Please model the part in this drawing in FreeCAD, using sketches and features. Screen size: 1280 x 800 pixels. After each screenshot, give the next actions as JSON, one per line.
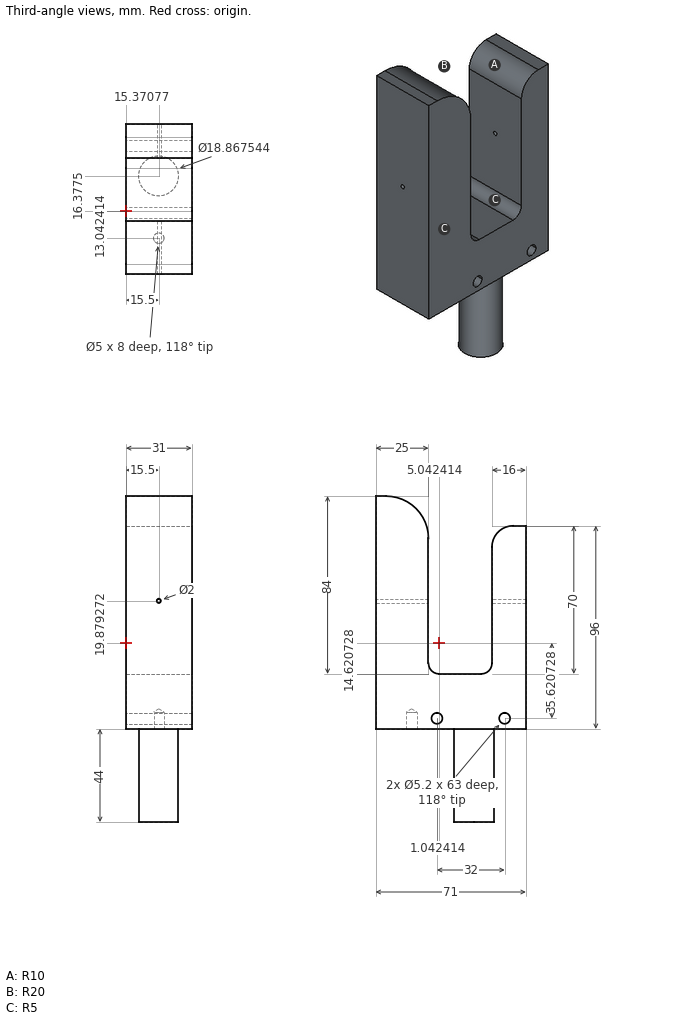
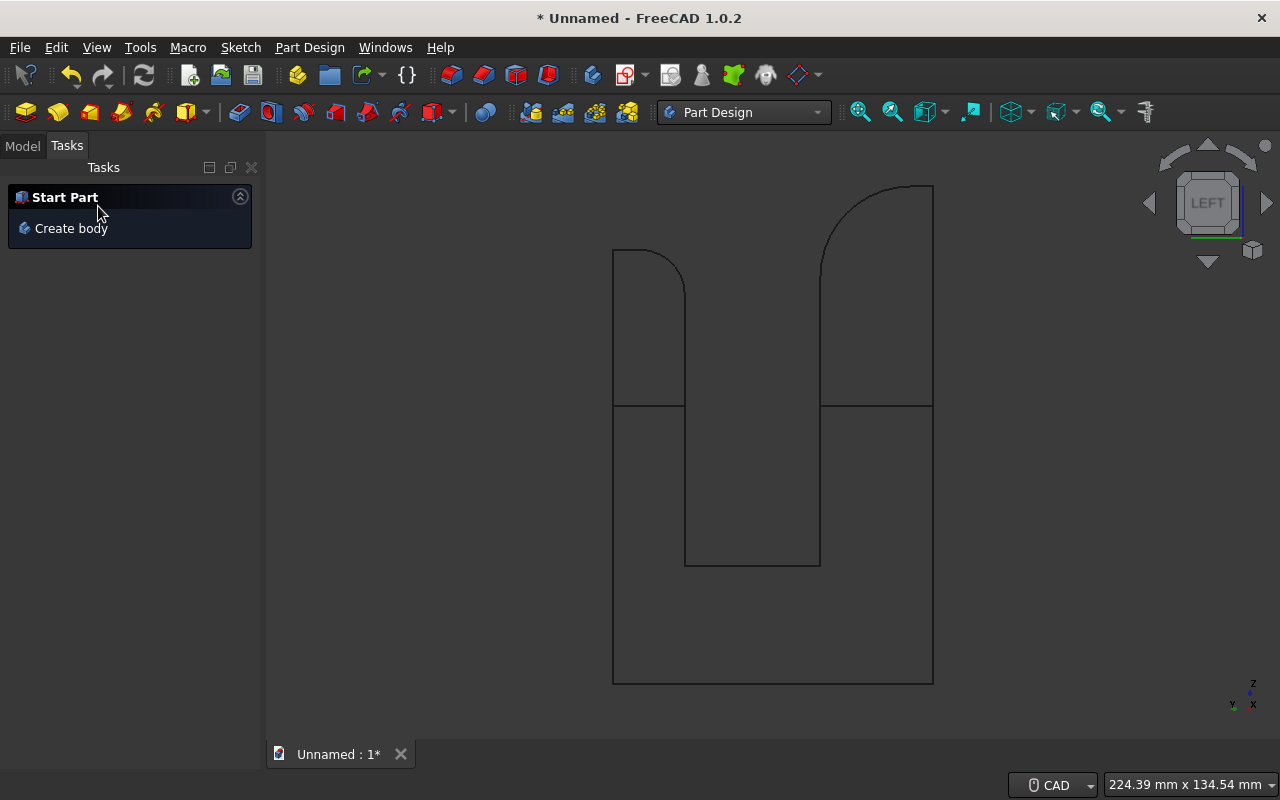
{"action": "key", "text": "0"}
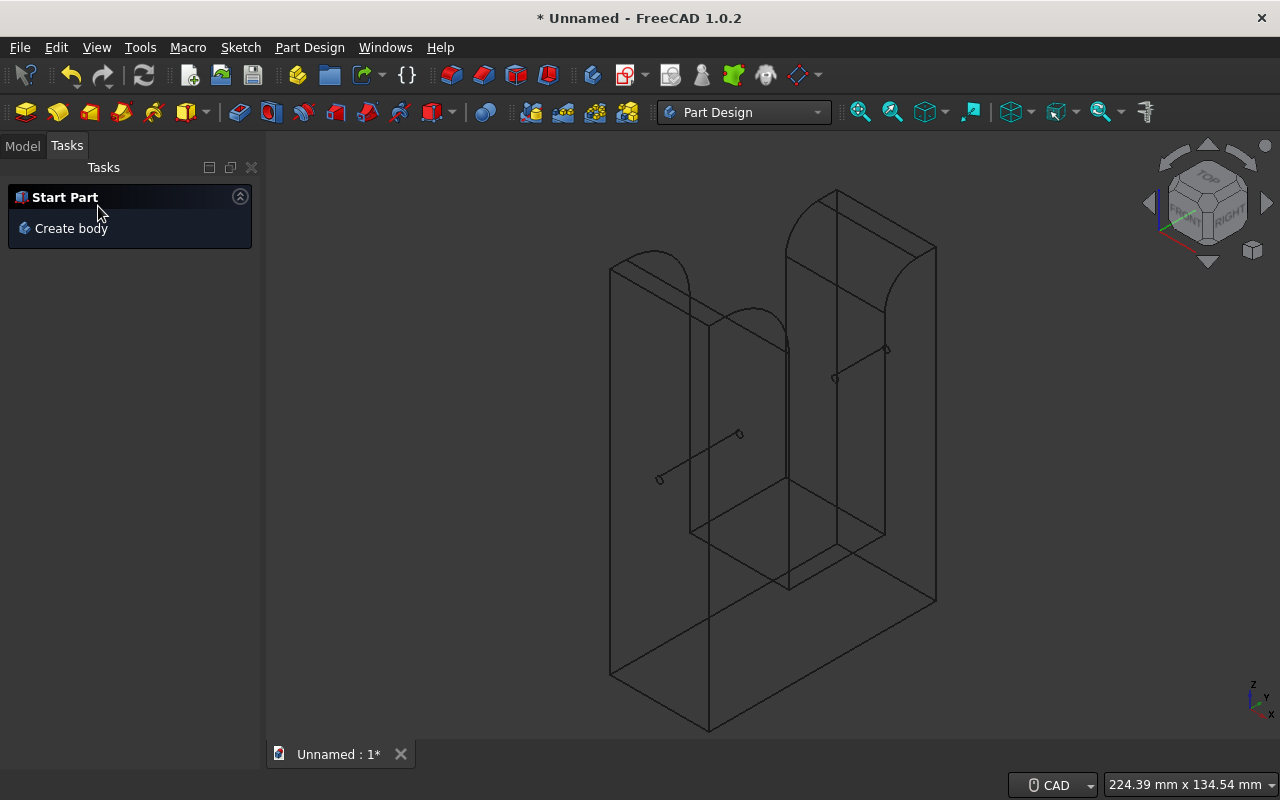
{"action": "left_click", "coordinate": [739, 560]}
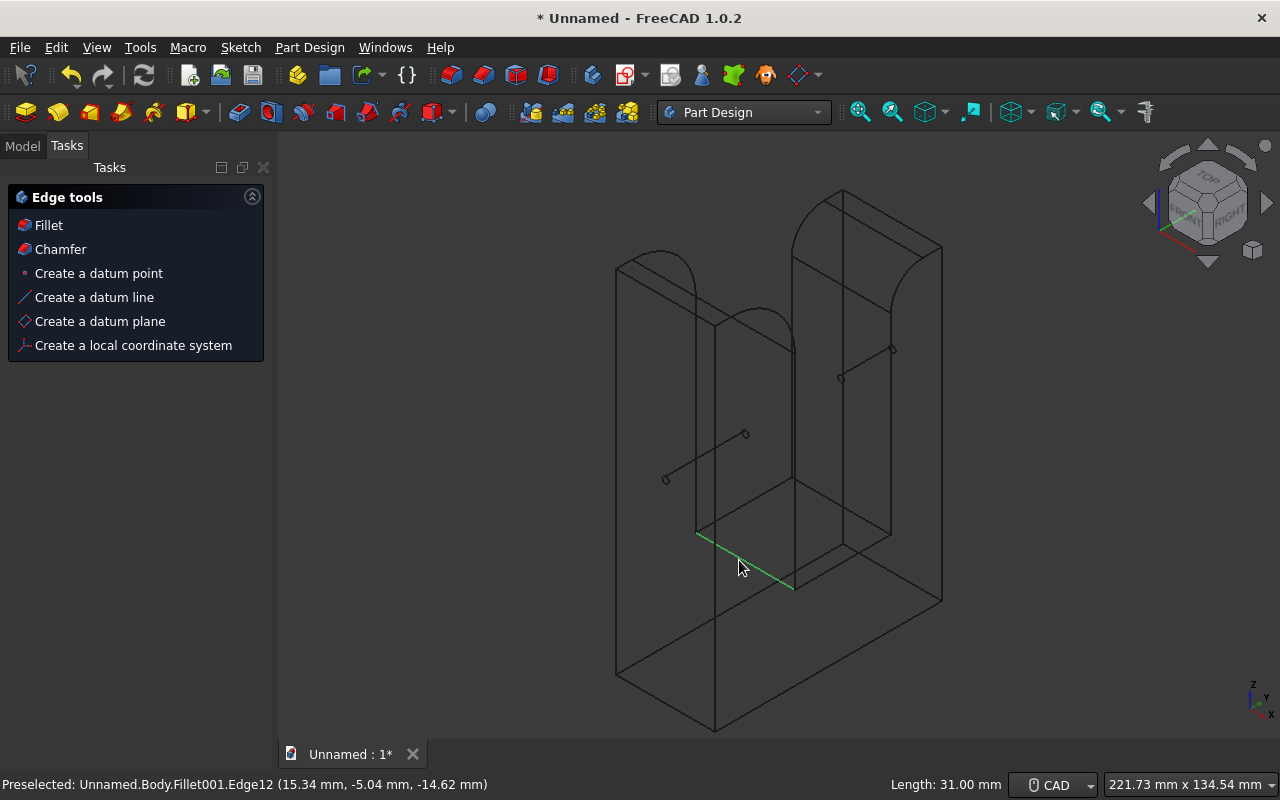
{"action": "left_click", "coordinate": [841, 505], "text": "ctrl"}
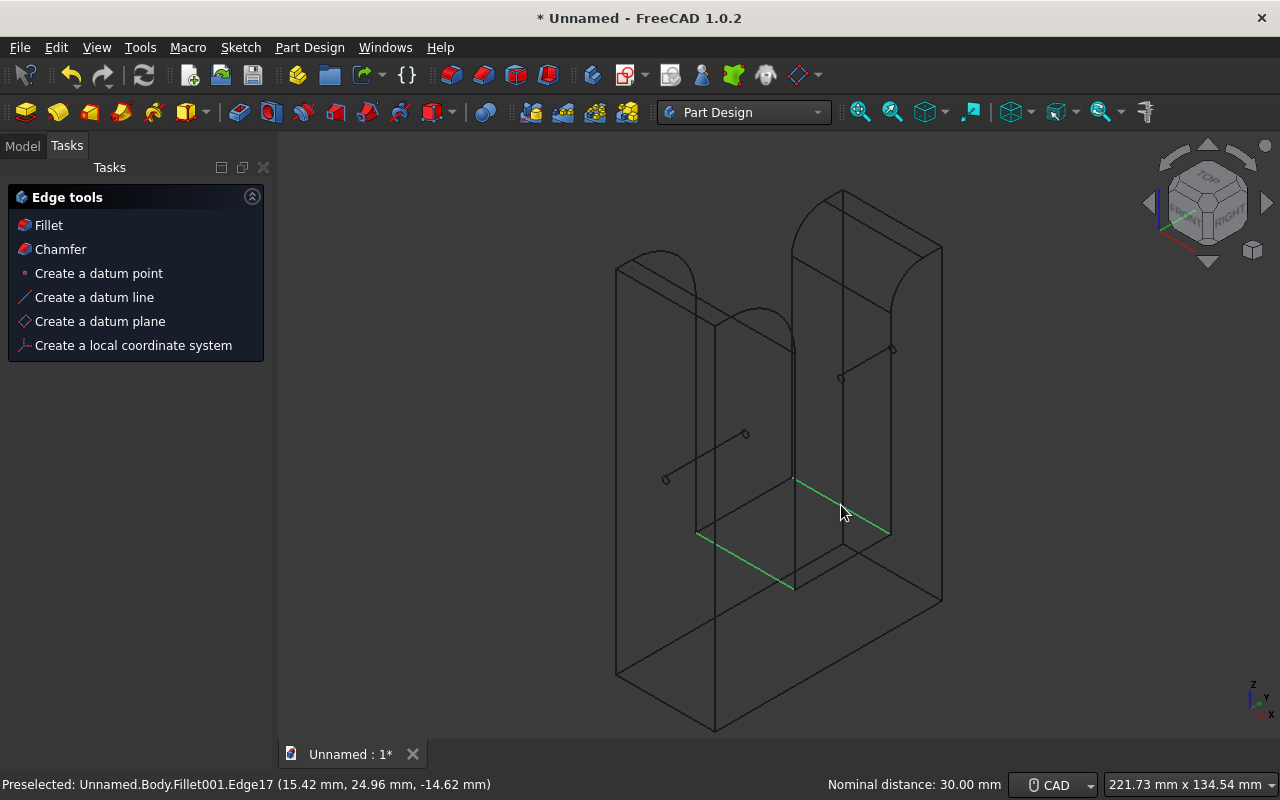
{"action": "key", "text": "v 1"}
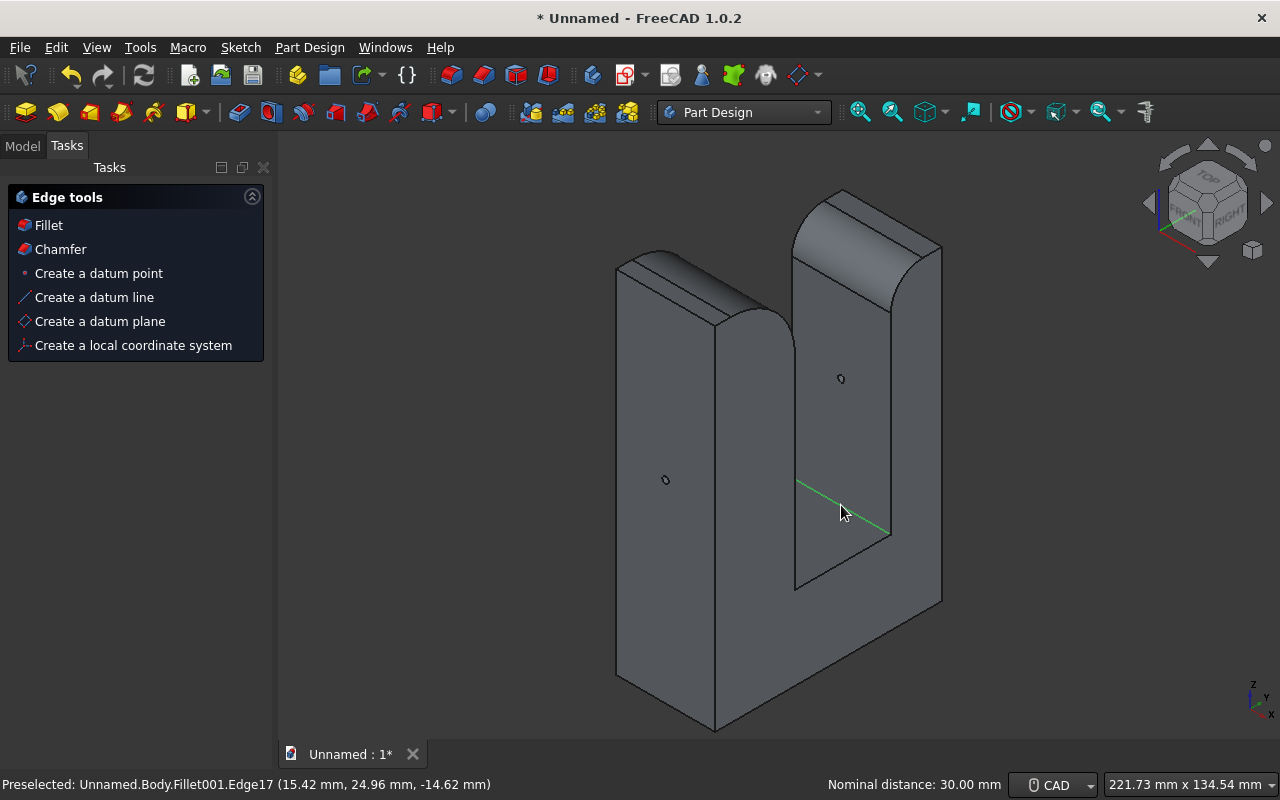
{"action": "left_click", "coordinate": [452, 76]}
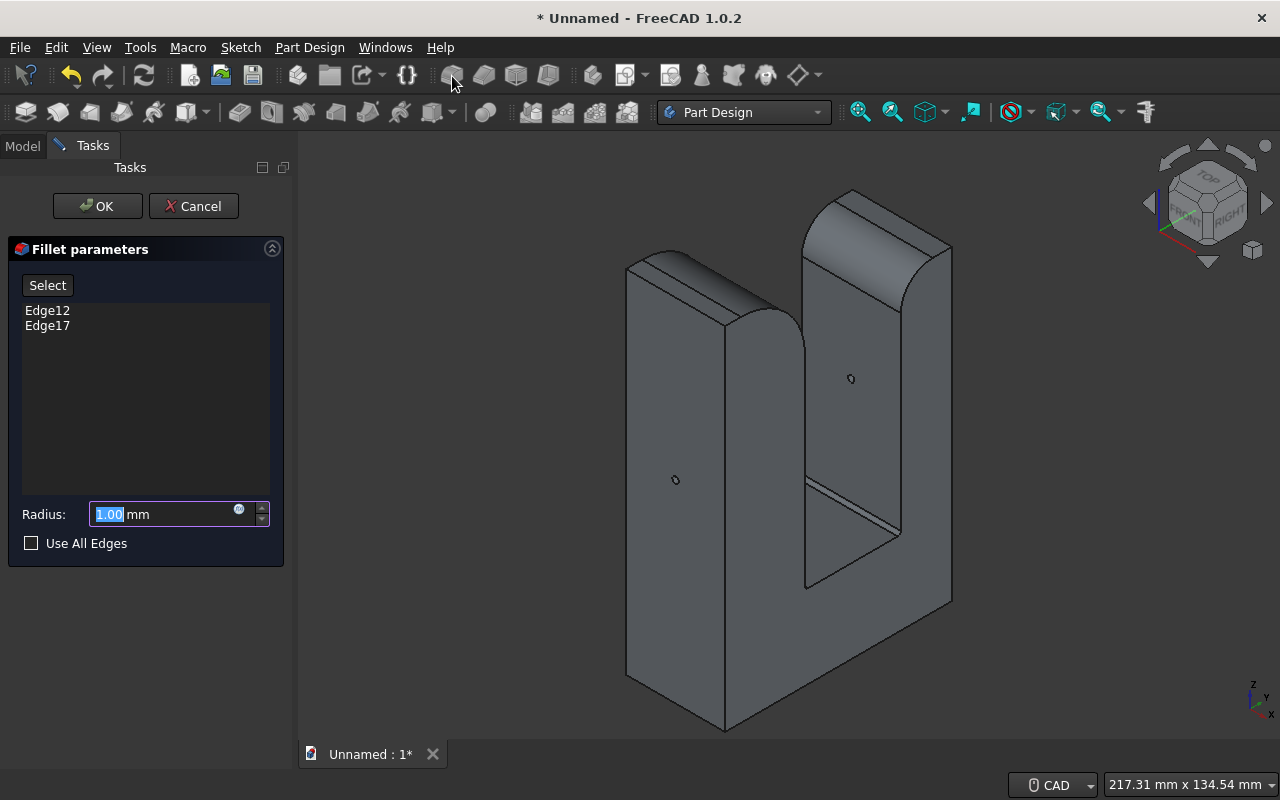
{"action": "type", "text": "5"}
{"action": "key", "text": "Tab"}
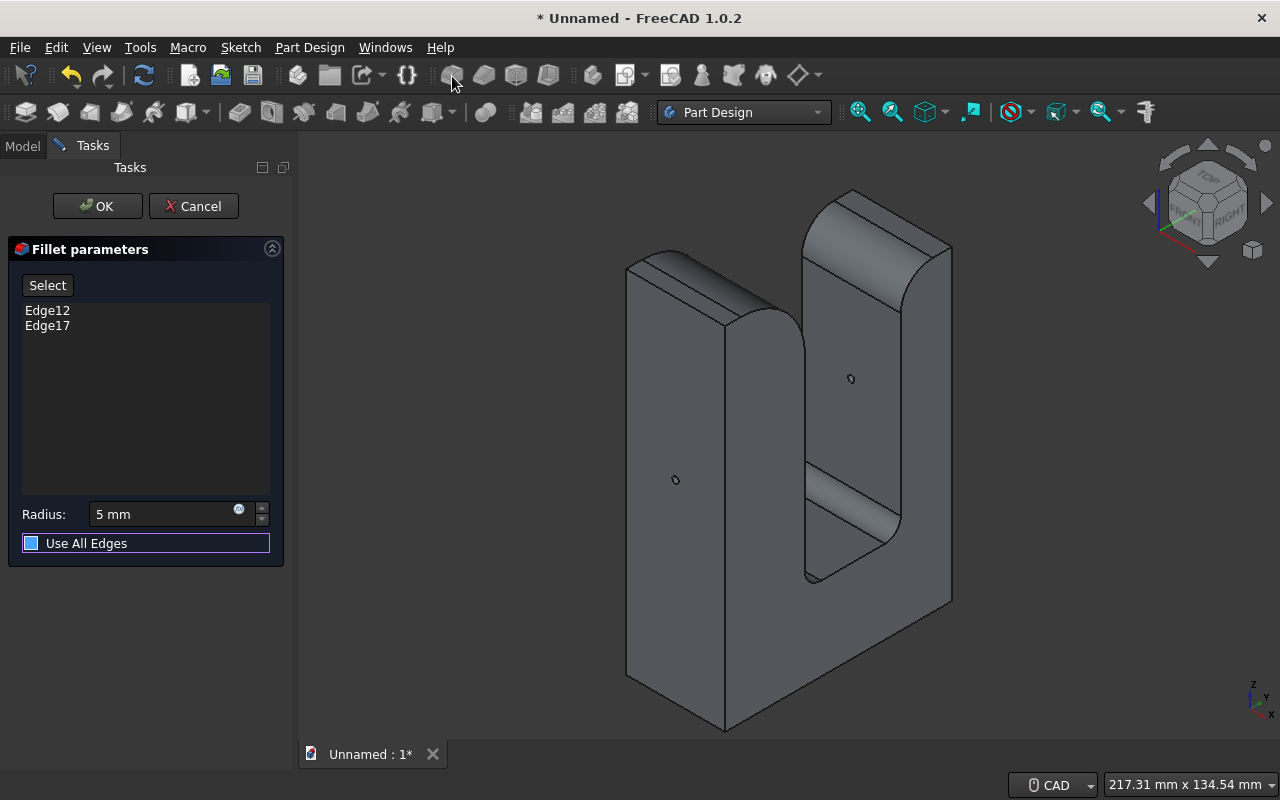
{"action": "left_click", "coordinate": [98, 206]}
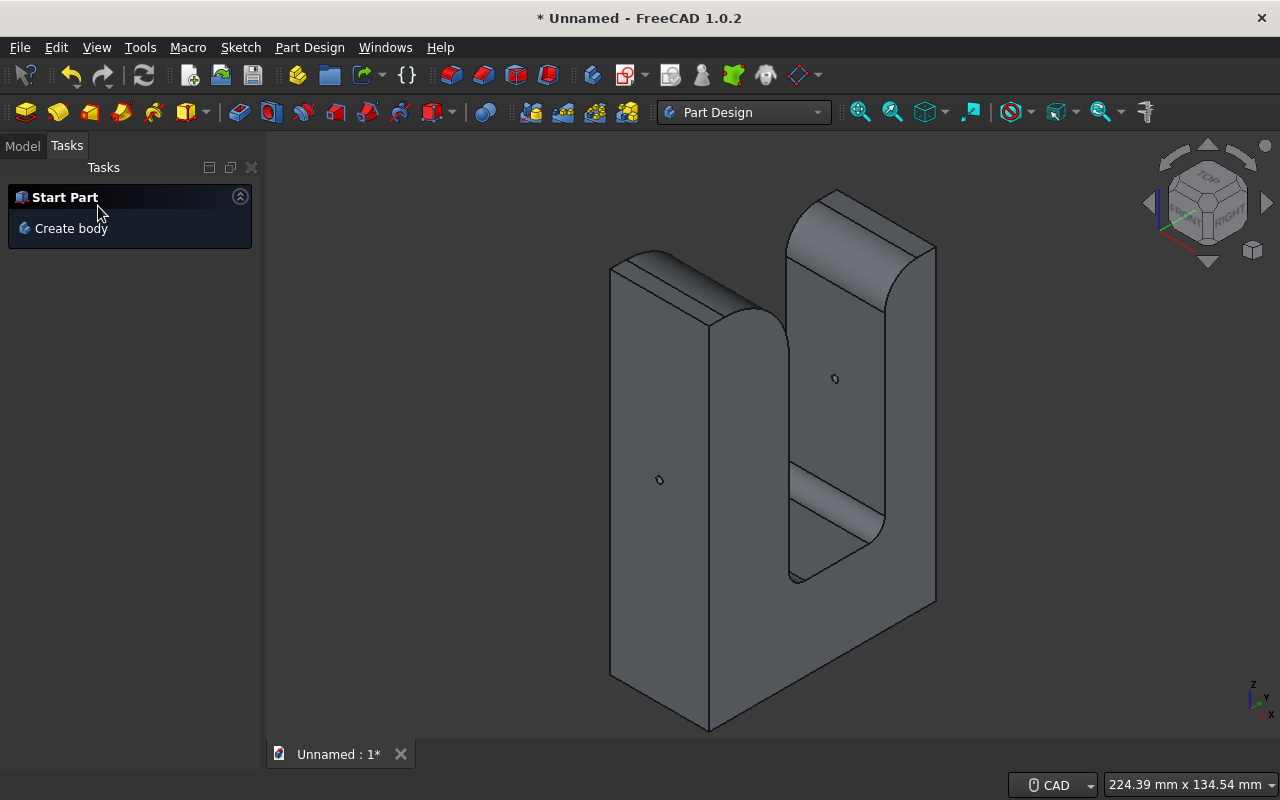
{"action": "left_click", "coordinate": [758, 616]}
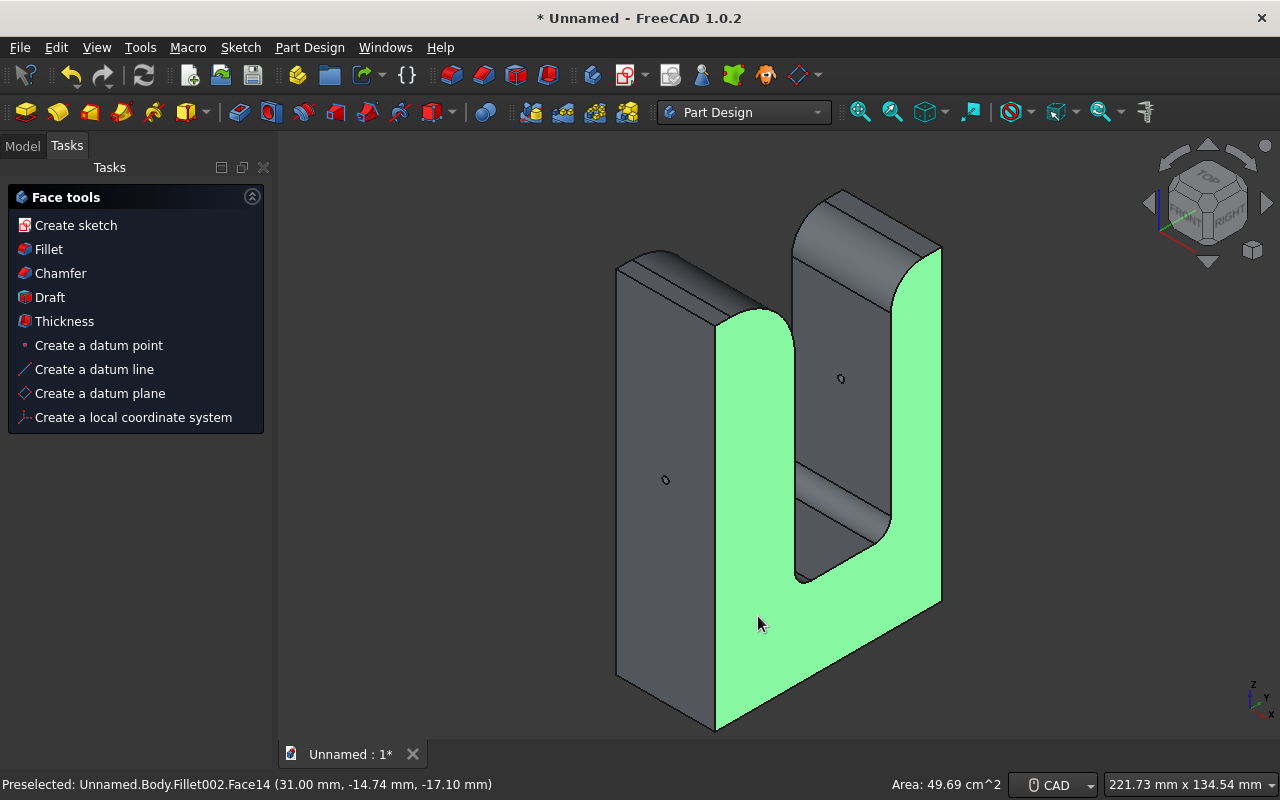
{"action": "left_click", "coordinate": [626, 76]}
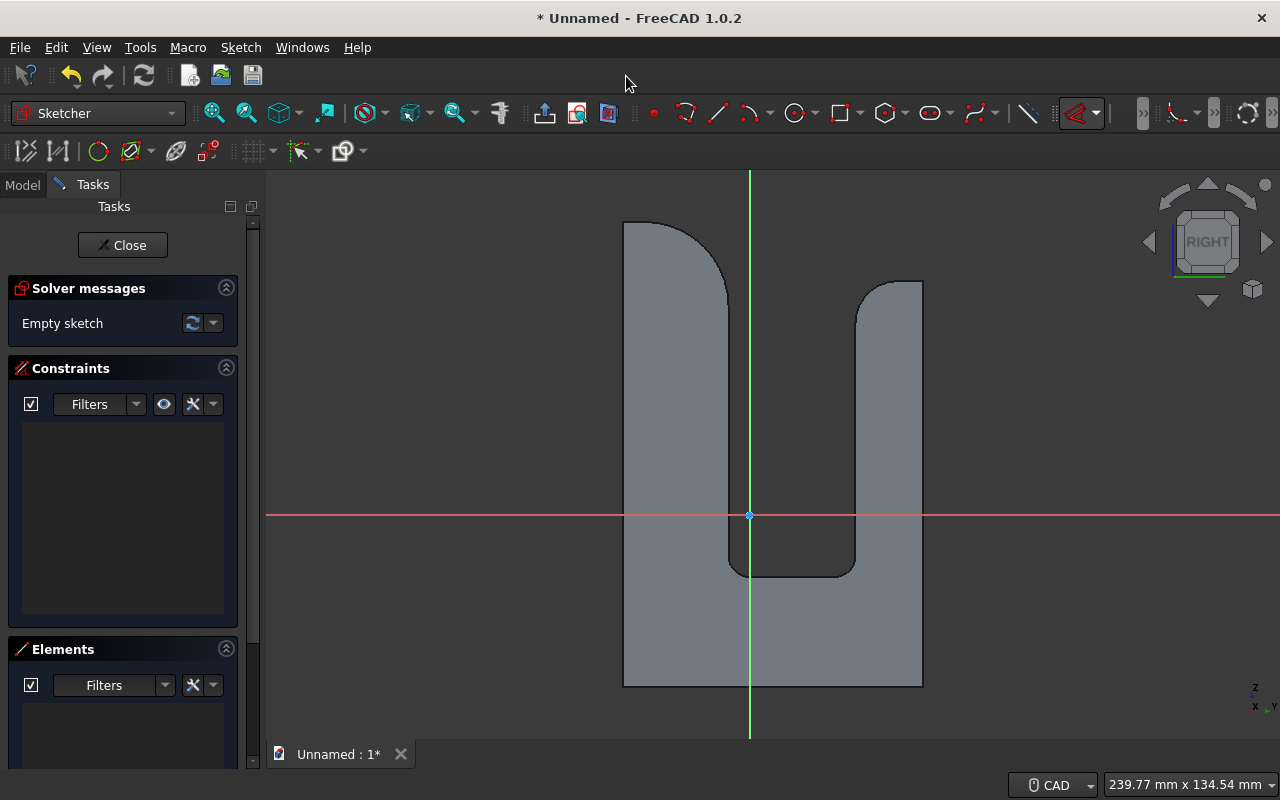
{"action": "scroll", "coordinate": [902, 711], "scroll_direction": "up", "scroll_amount": 4}